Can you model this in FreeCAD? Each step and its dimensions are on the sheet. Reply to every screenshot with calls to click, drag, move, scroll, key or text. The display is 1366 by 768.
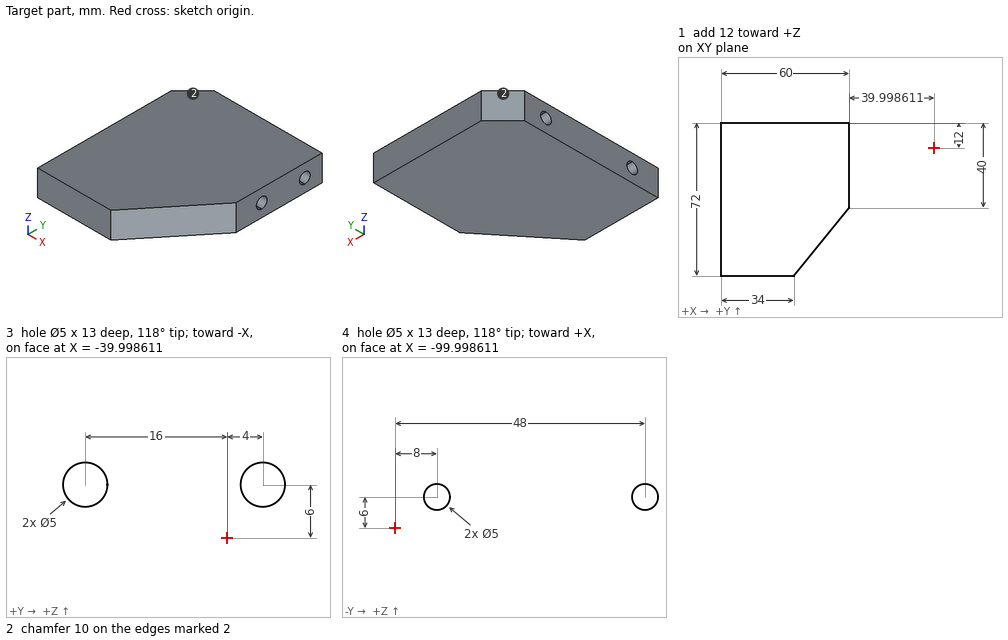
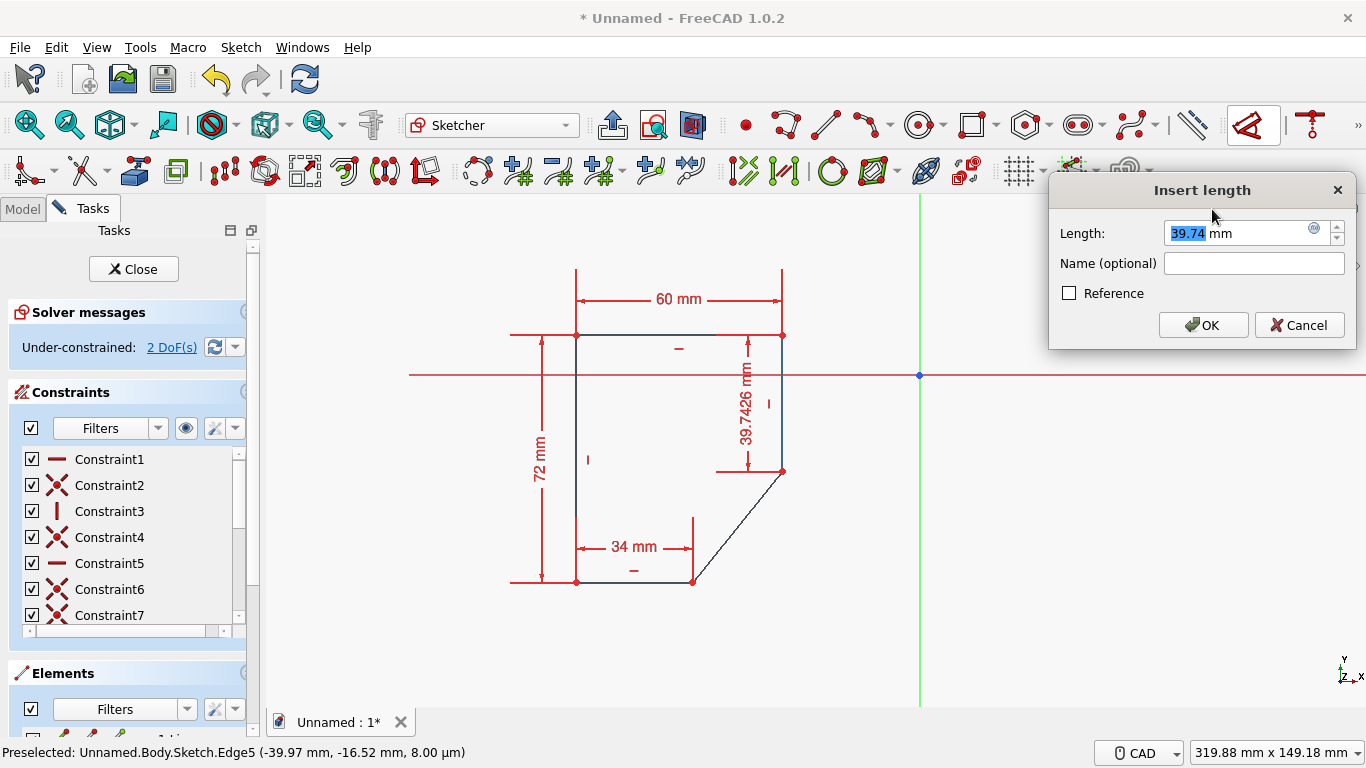
text(40)
key(Return)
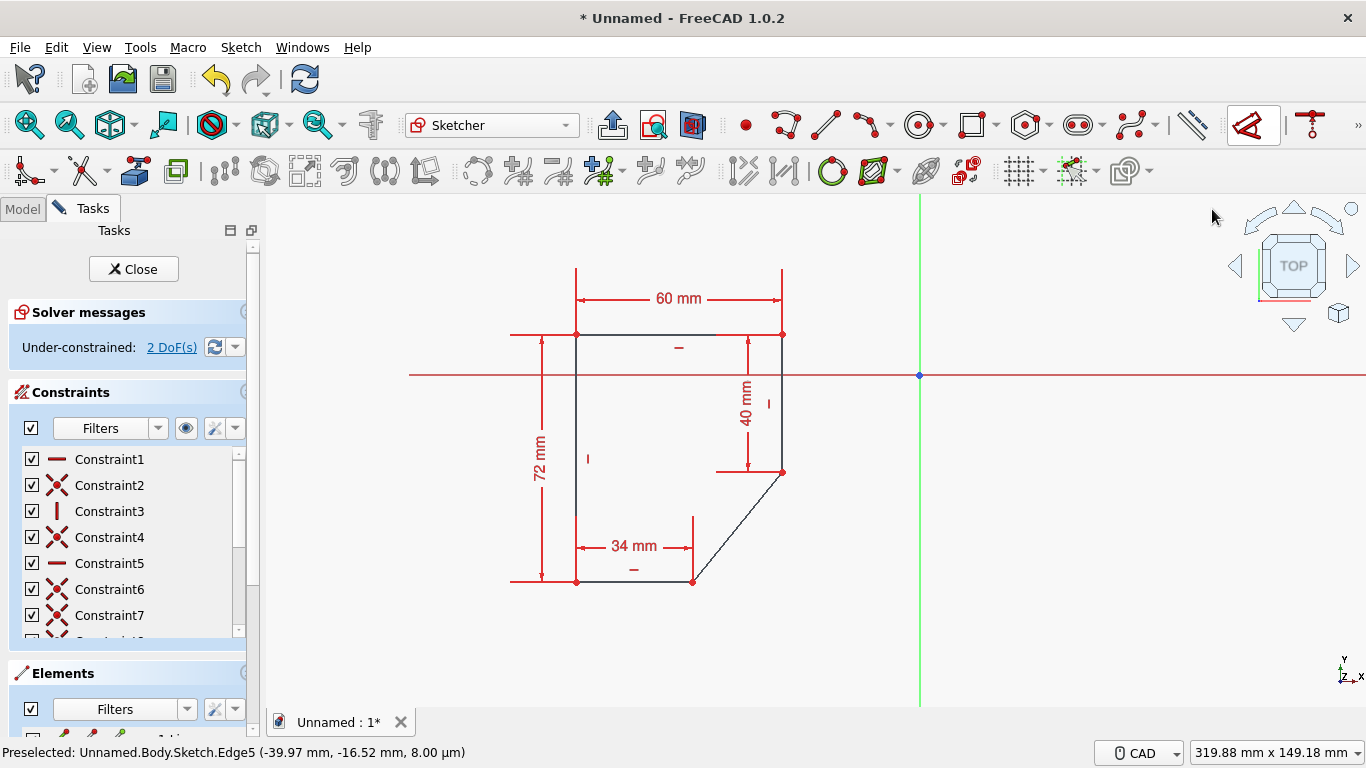
click(782, 335)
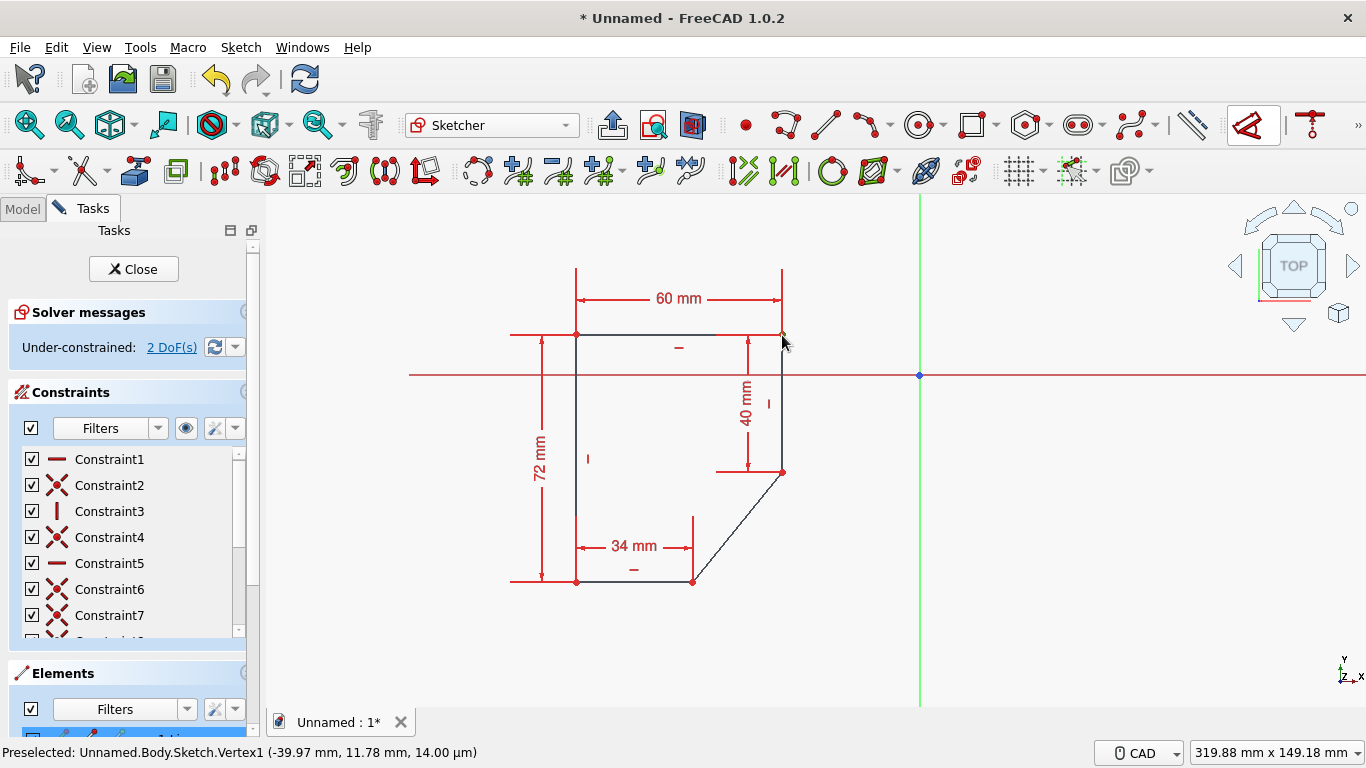
click(1274, 126)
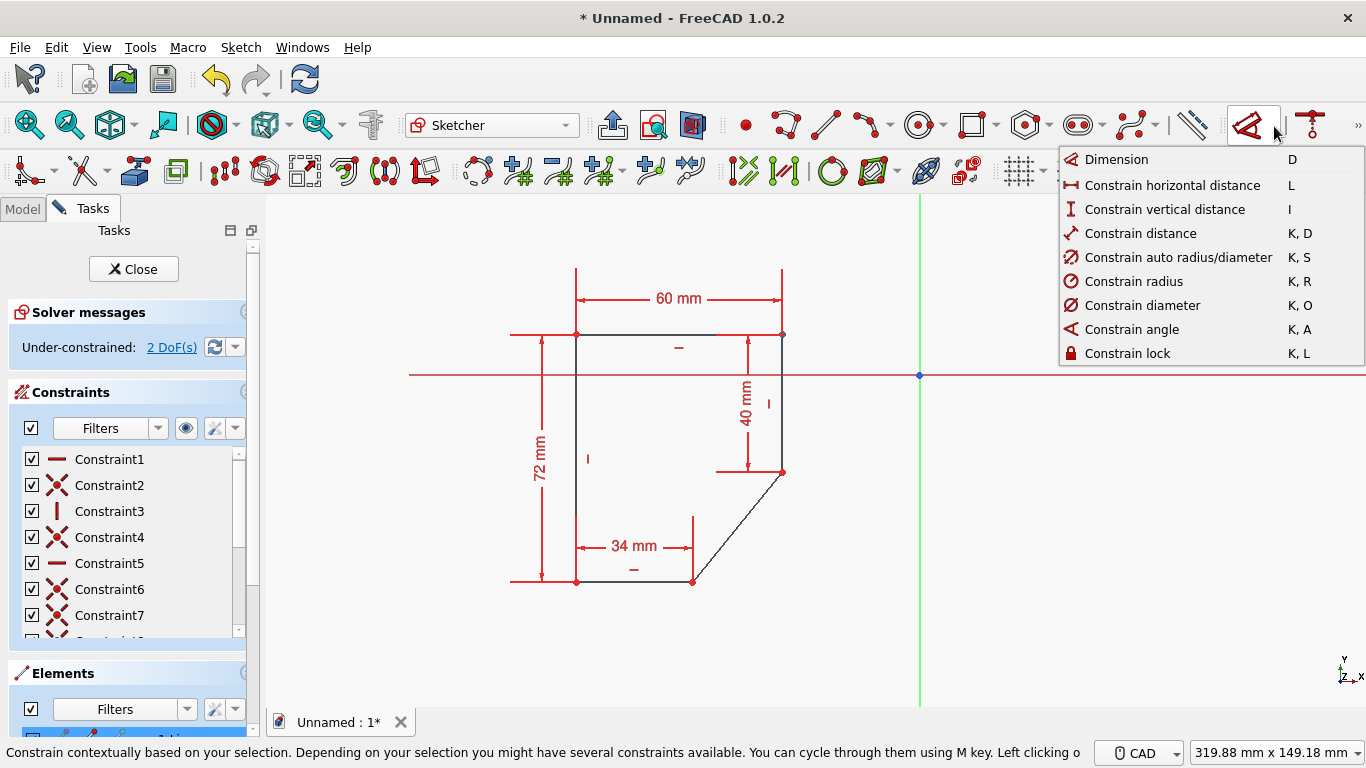
click(1212, 209)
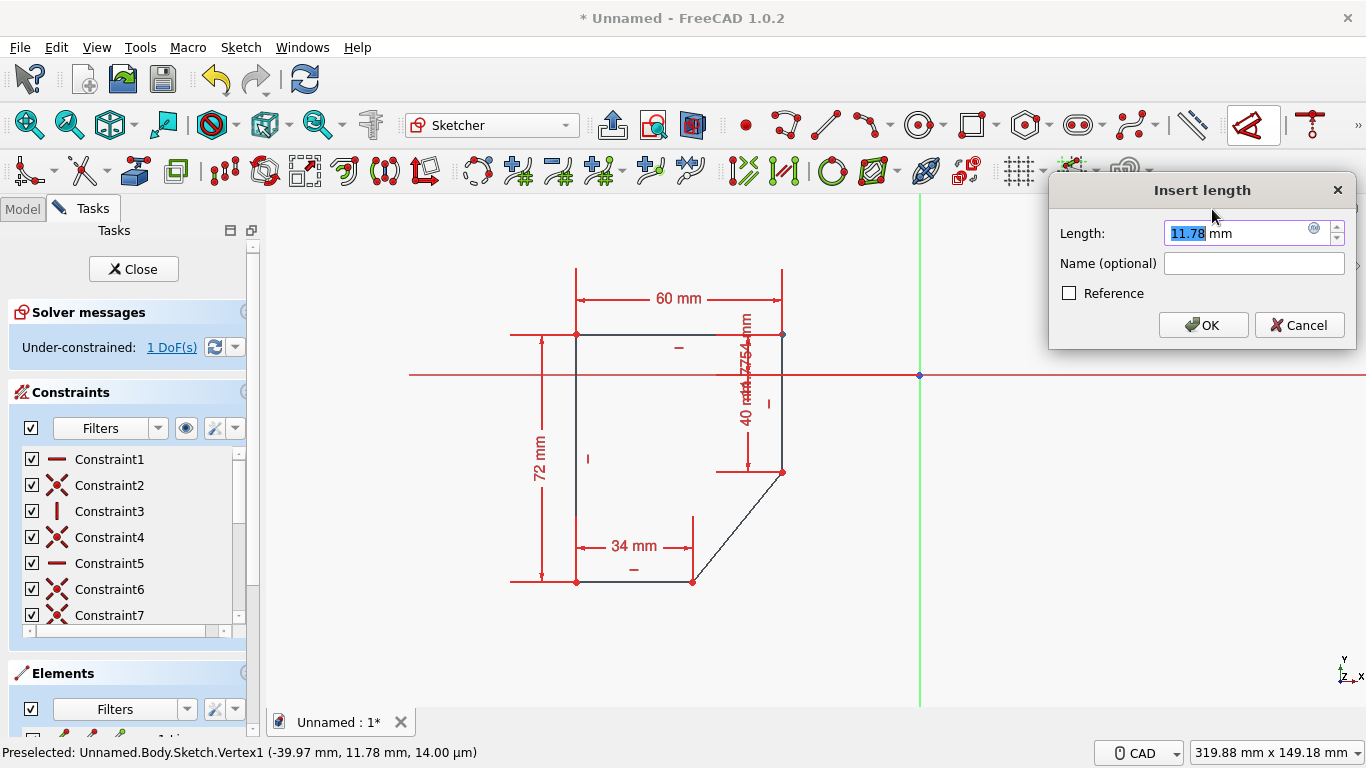
text(12)
key(Return)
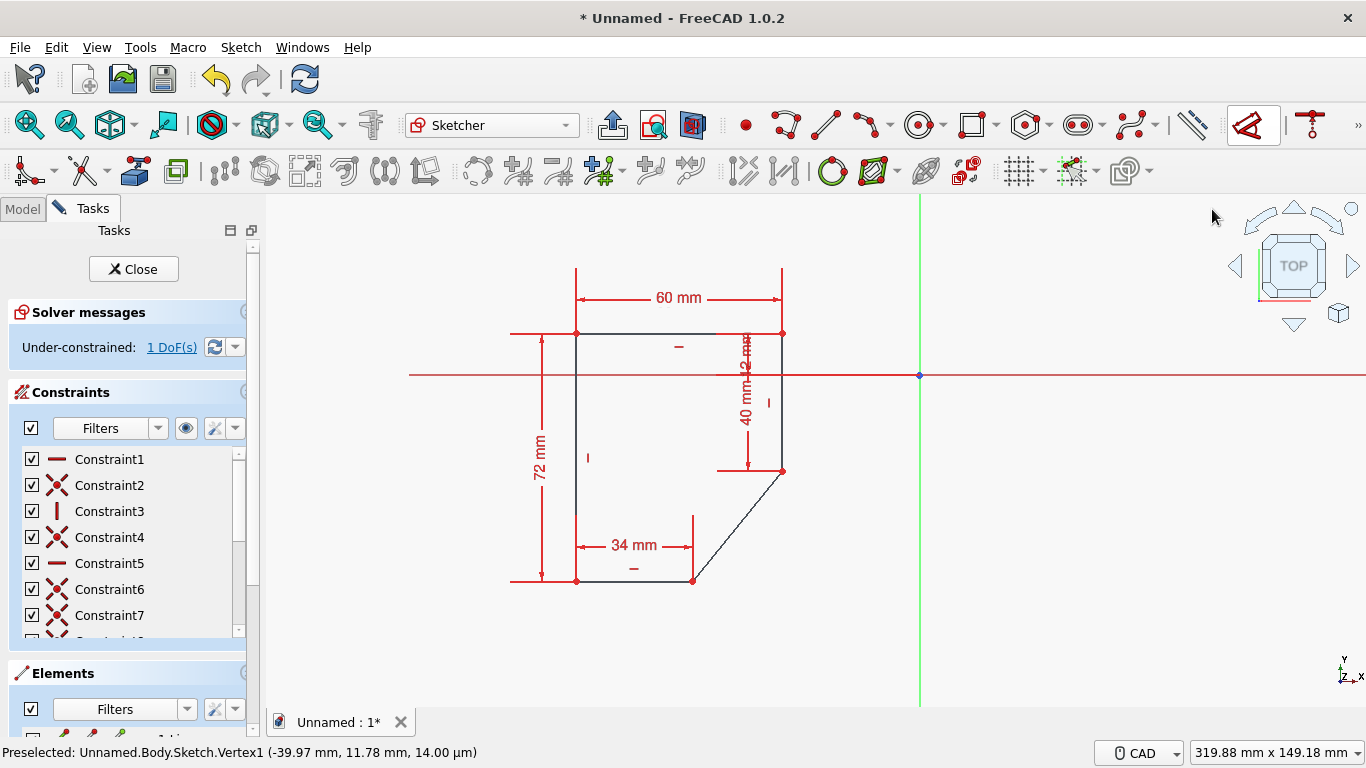
click(782, 334)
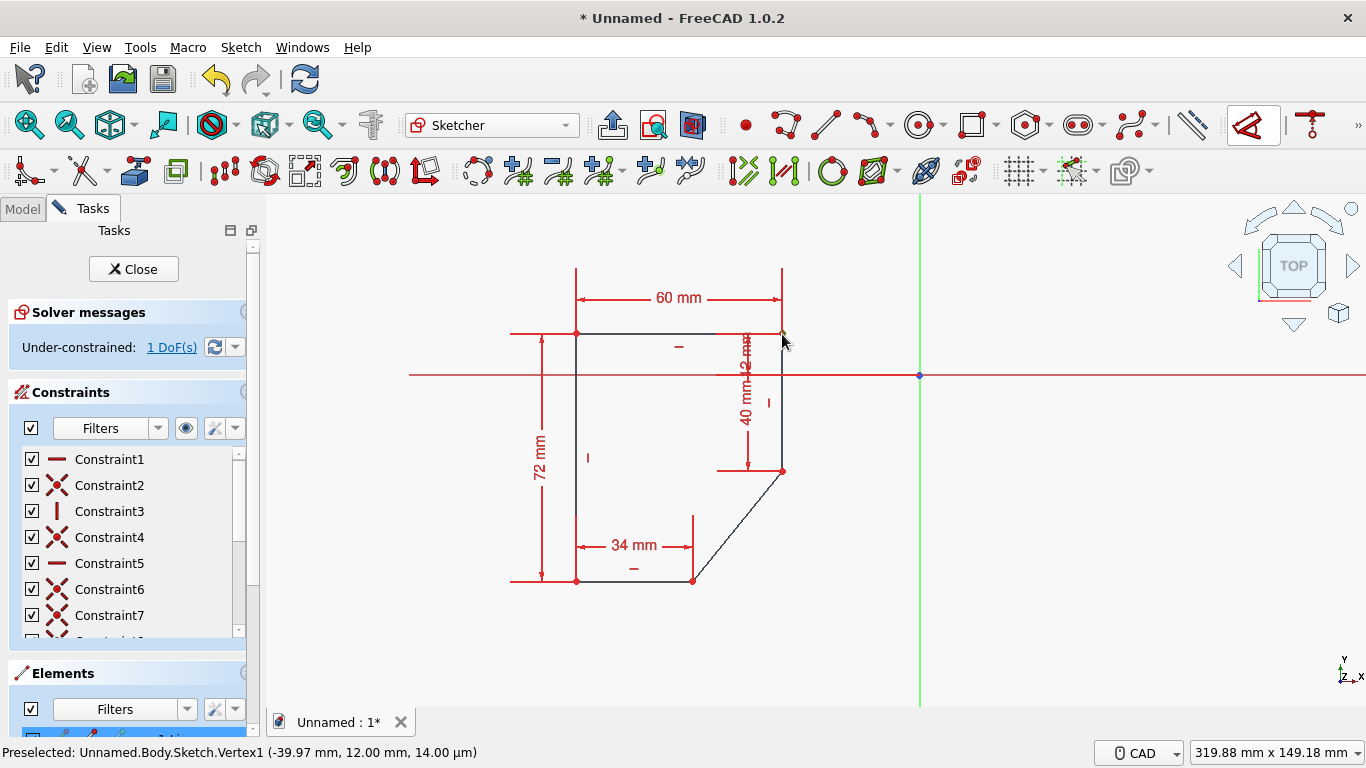
key(l)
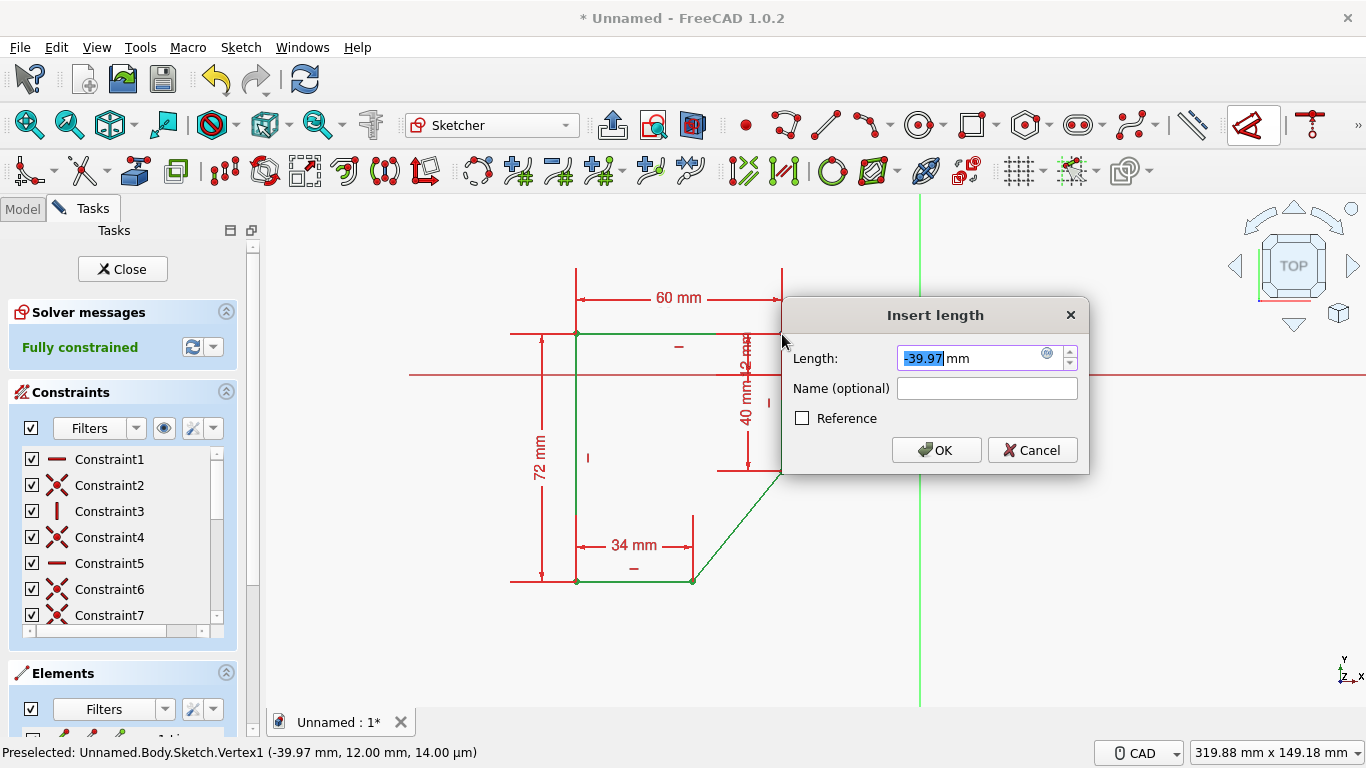
text(-39.998611)
key(Return)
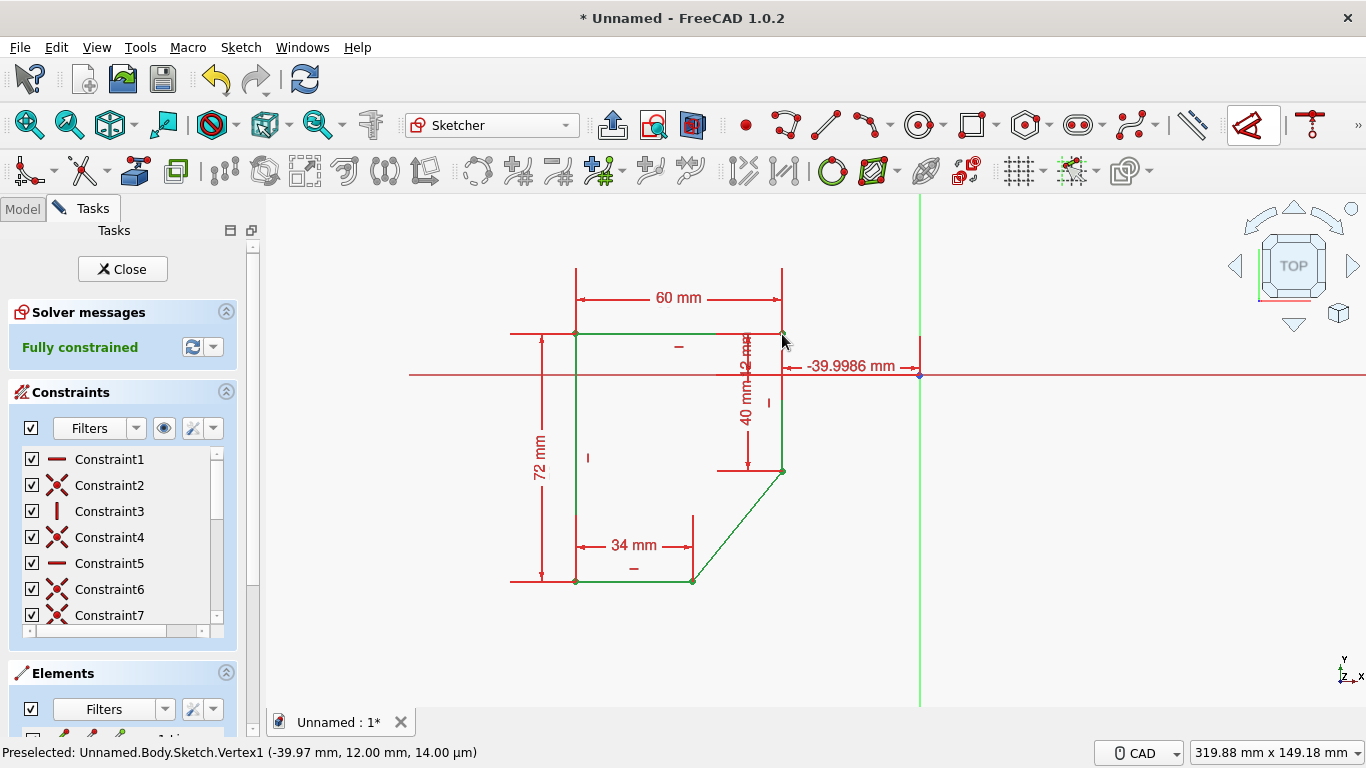
click(123, 269)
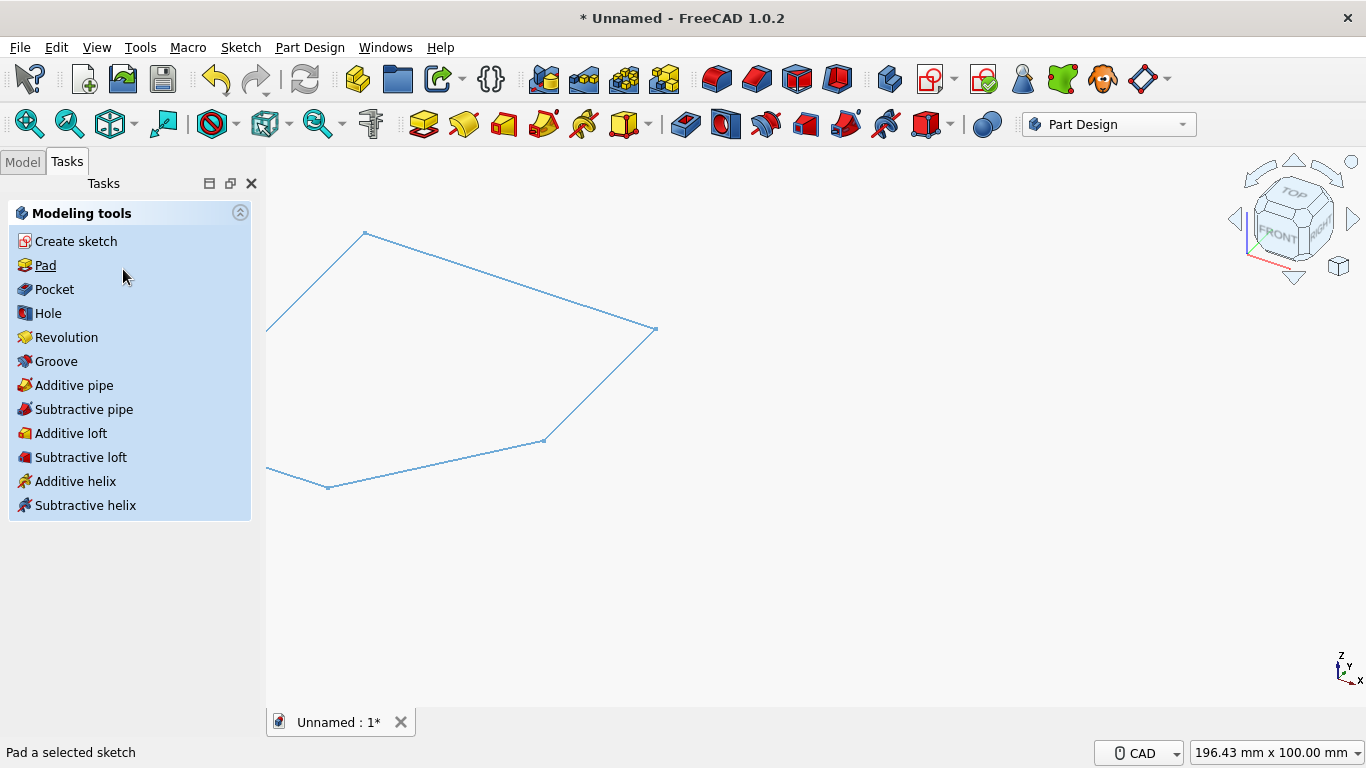
click(424, 124)